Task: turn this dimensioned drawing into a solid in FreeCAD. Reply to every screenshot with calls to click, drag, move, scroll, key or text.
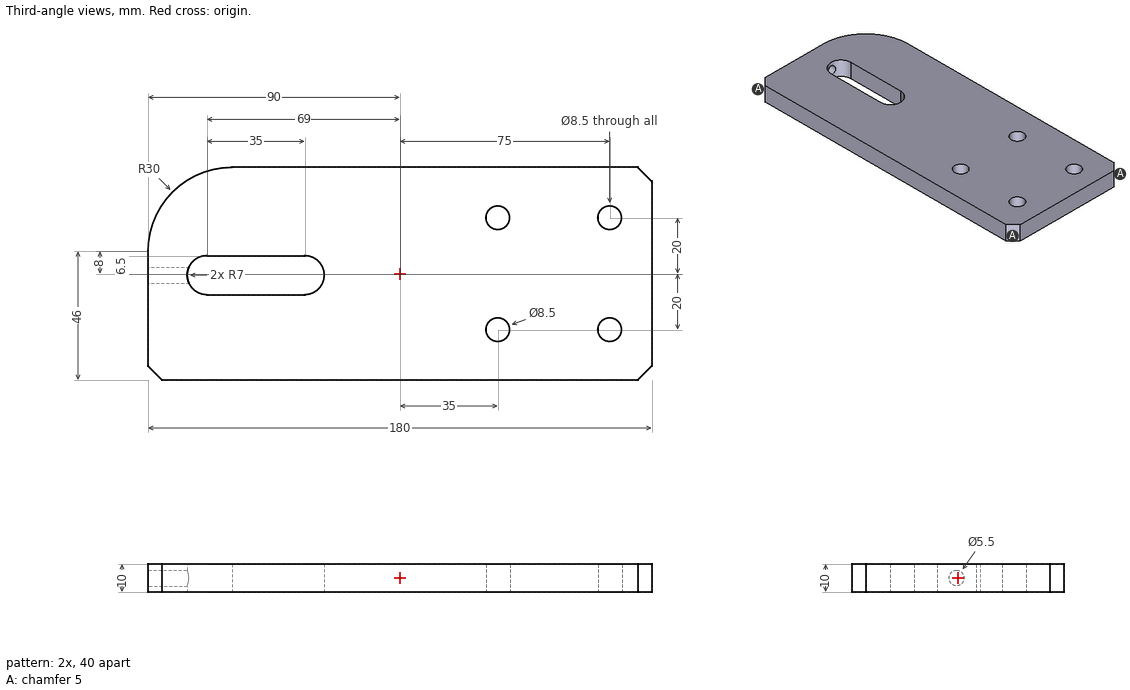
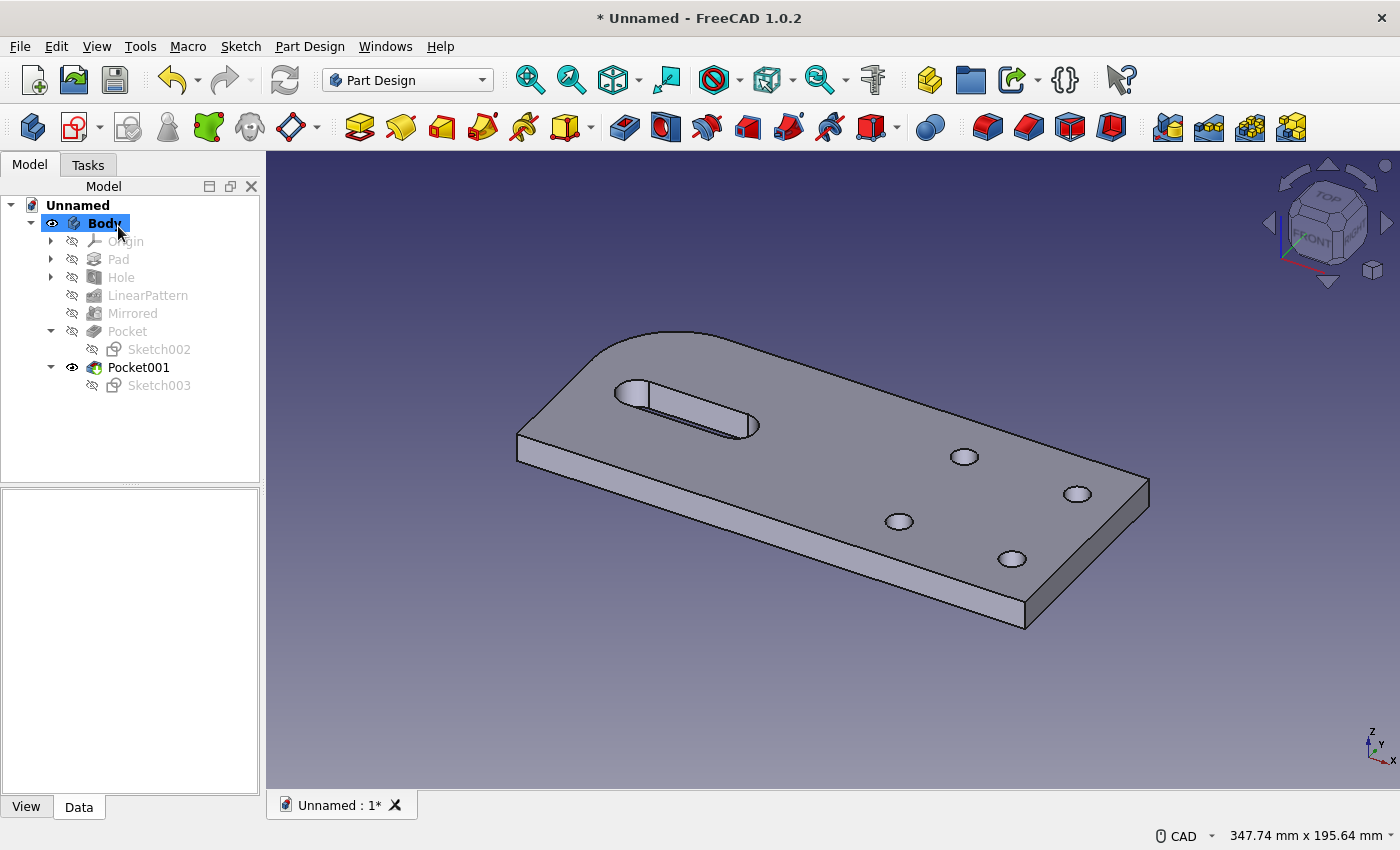
key(6)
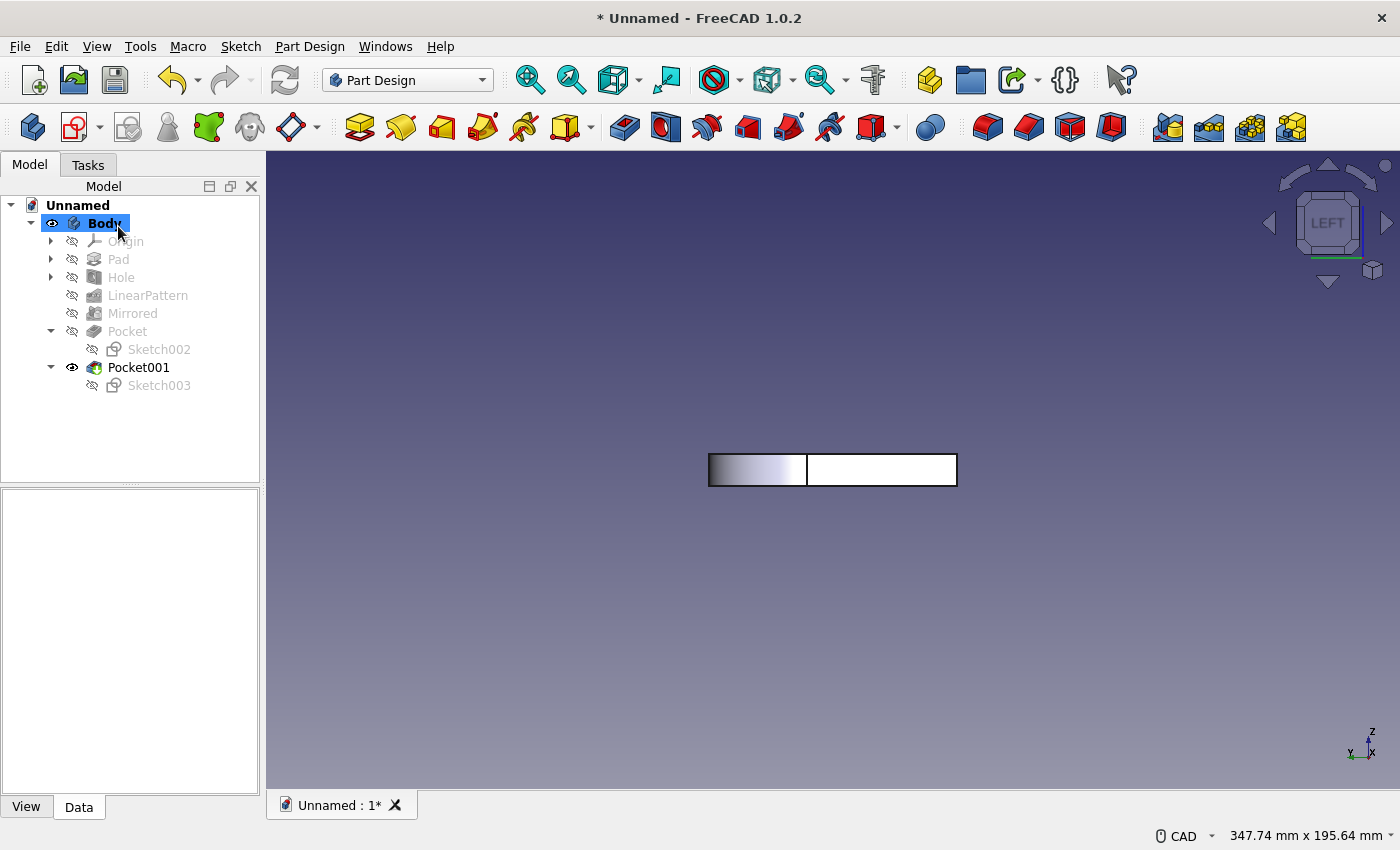
click(531, 80)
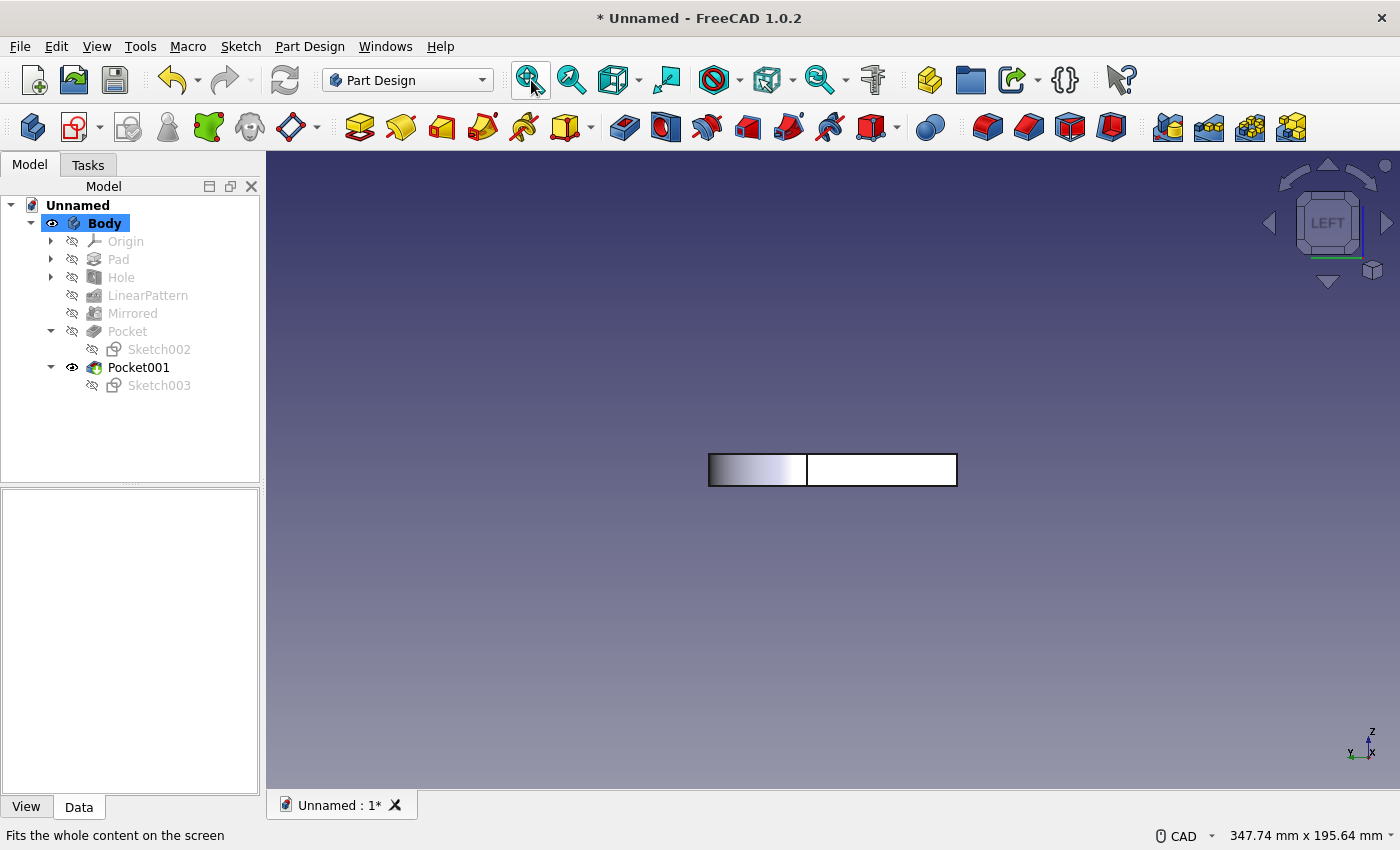
click(839, 469)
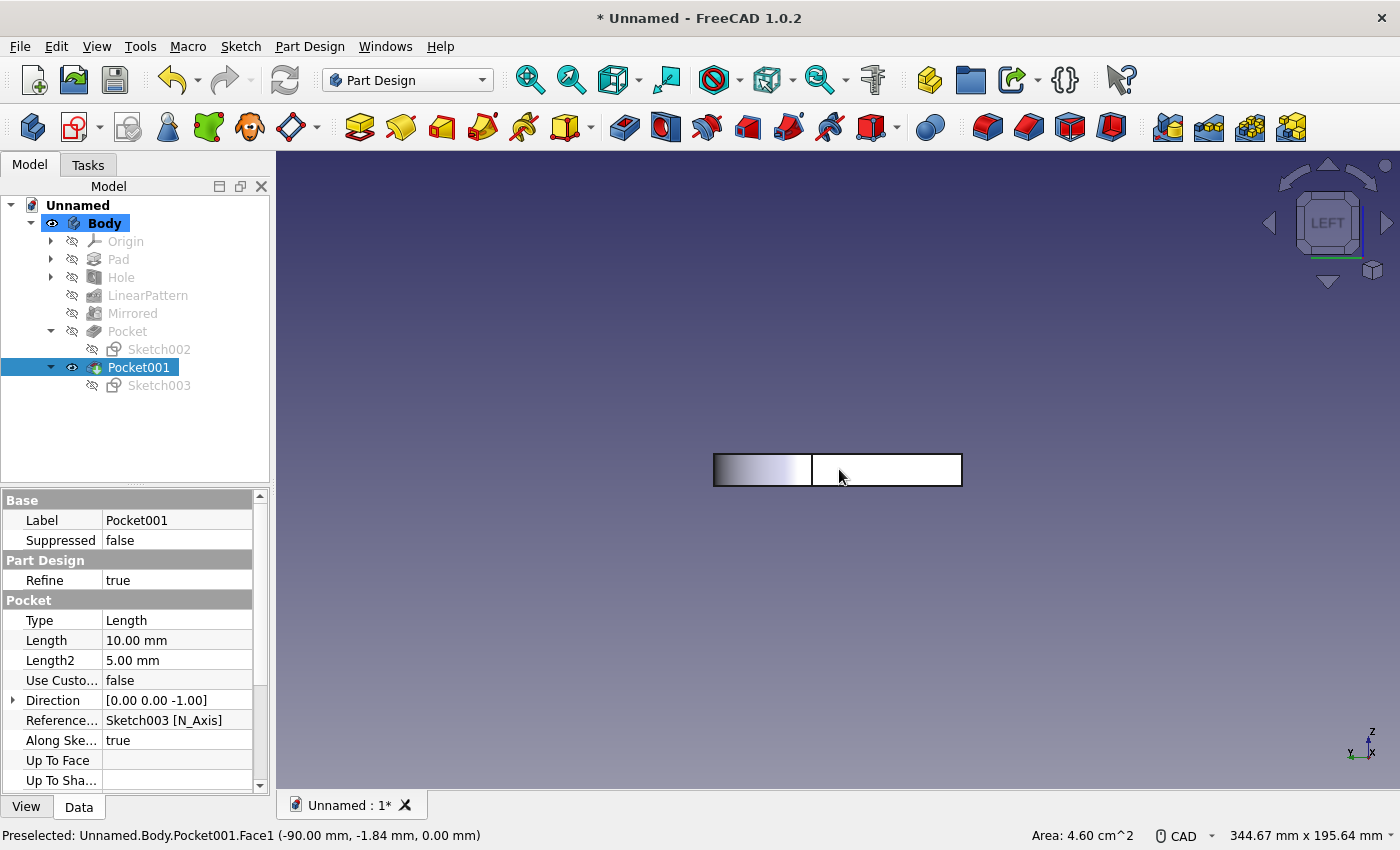
click(74, 128)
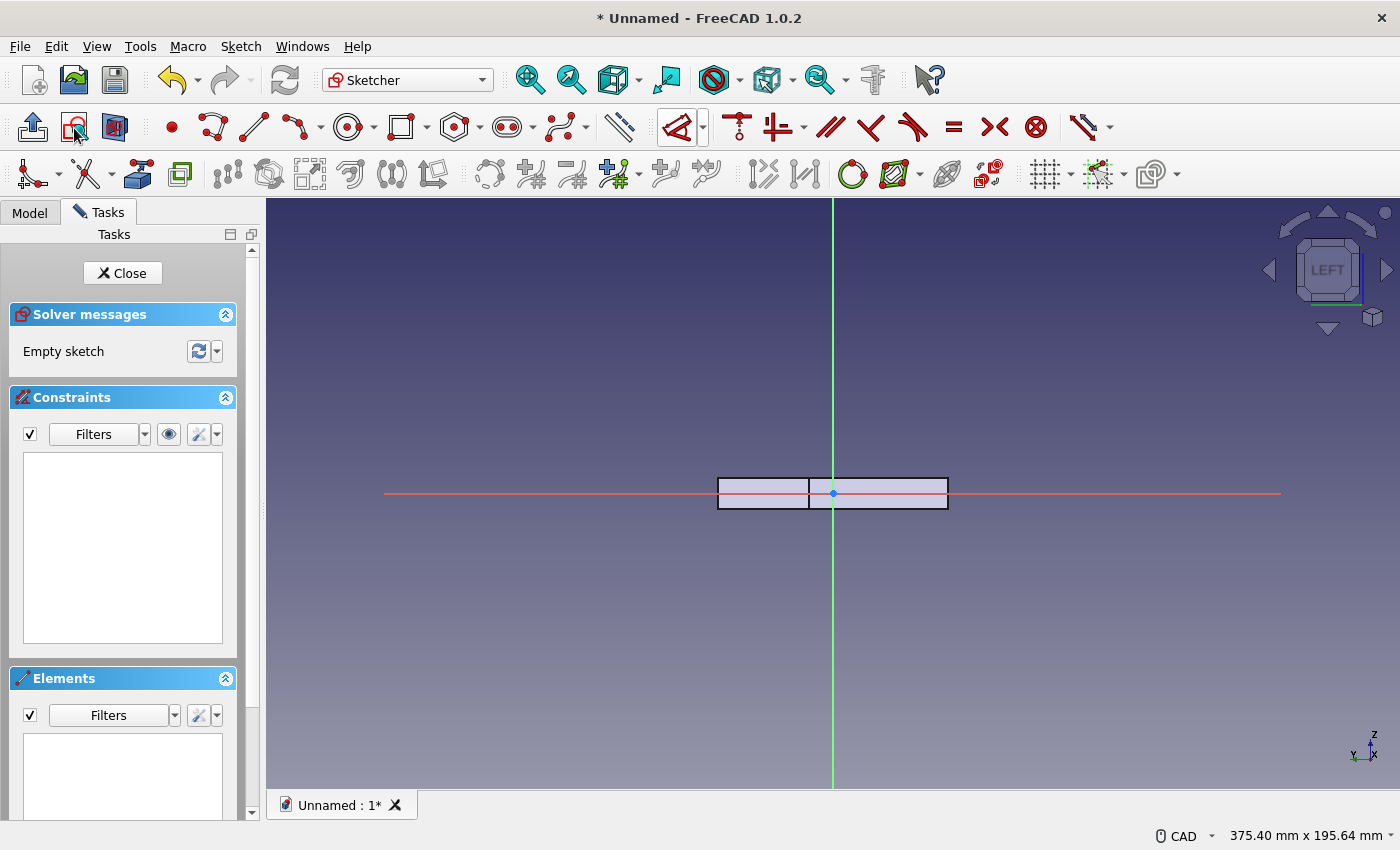
scroll(838, 494, up, 15)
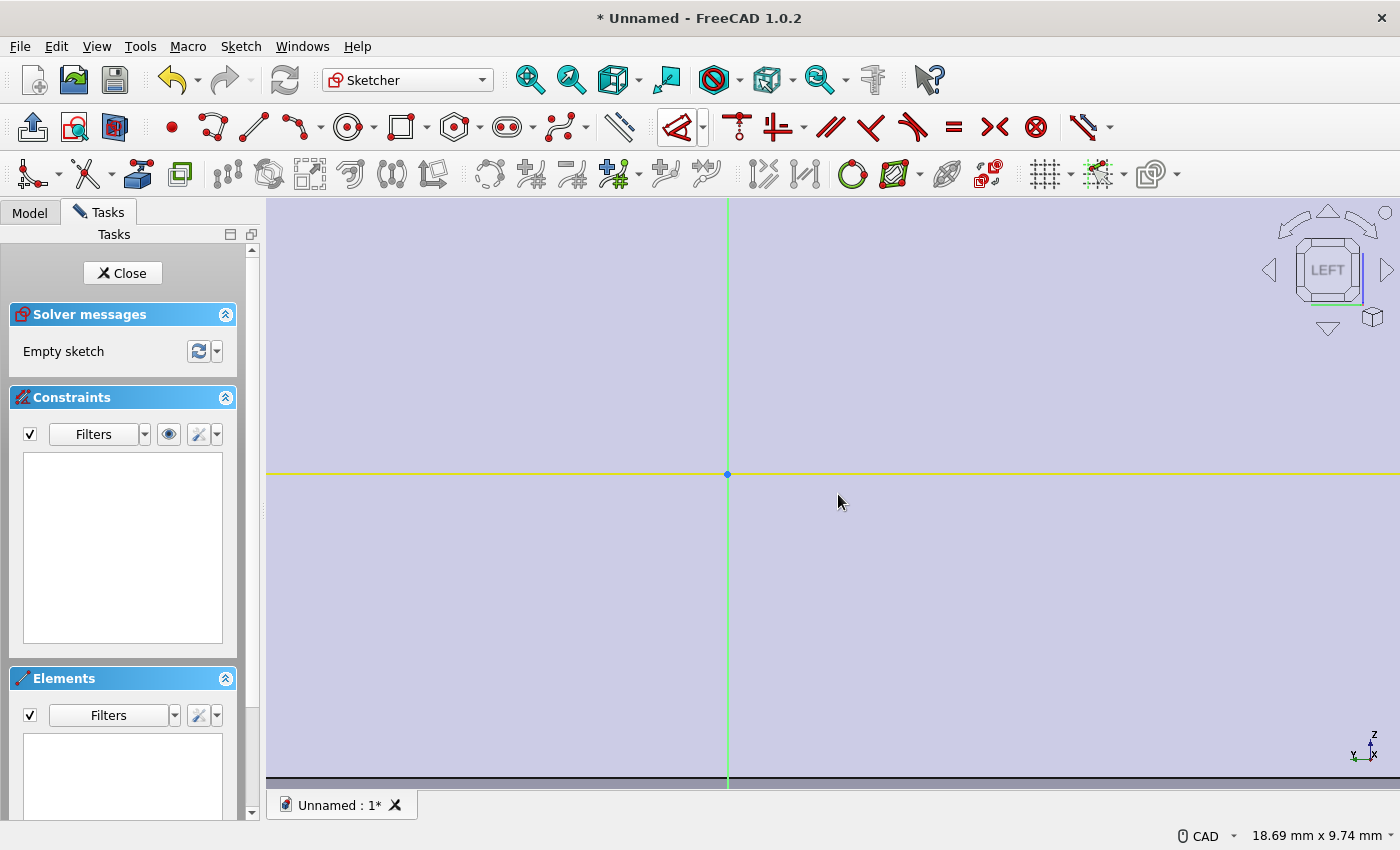
click(348, 128)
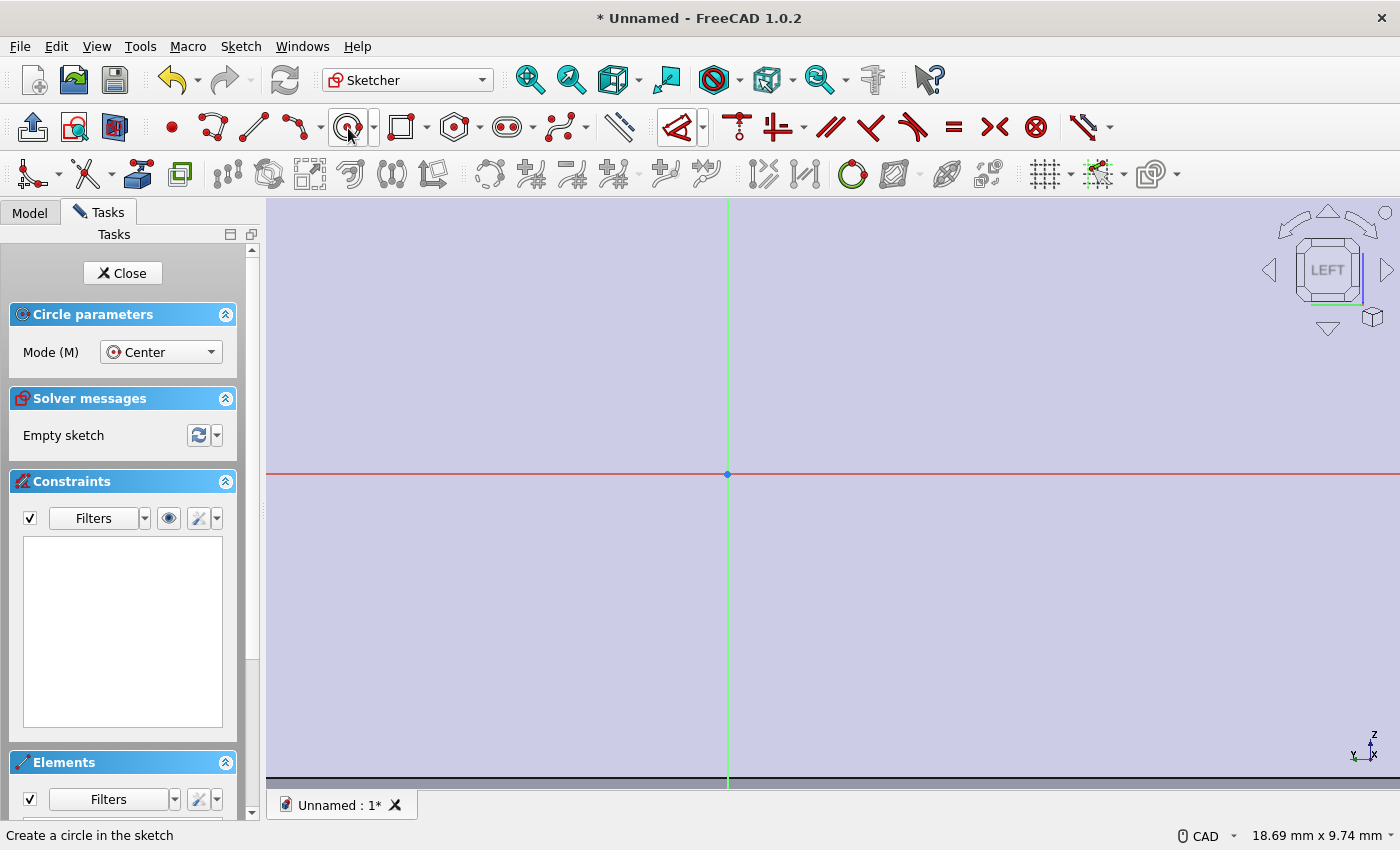
click(758, 474)
click(876, 356)
key(Escape)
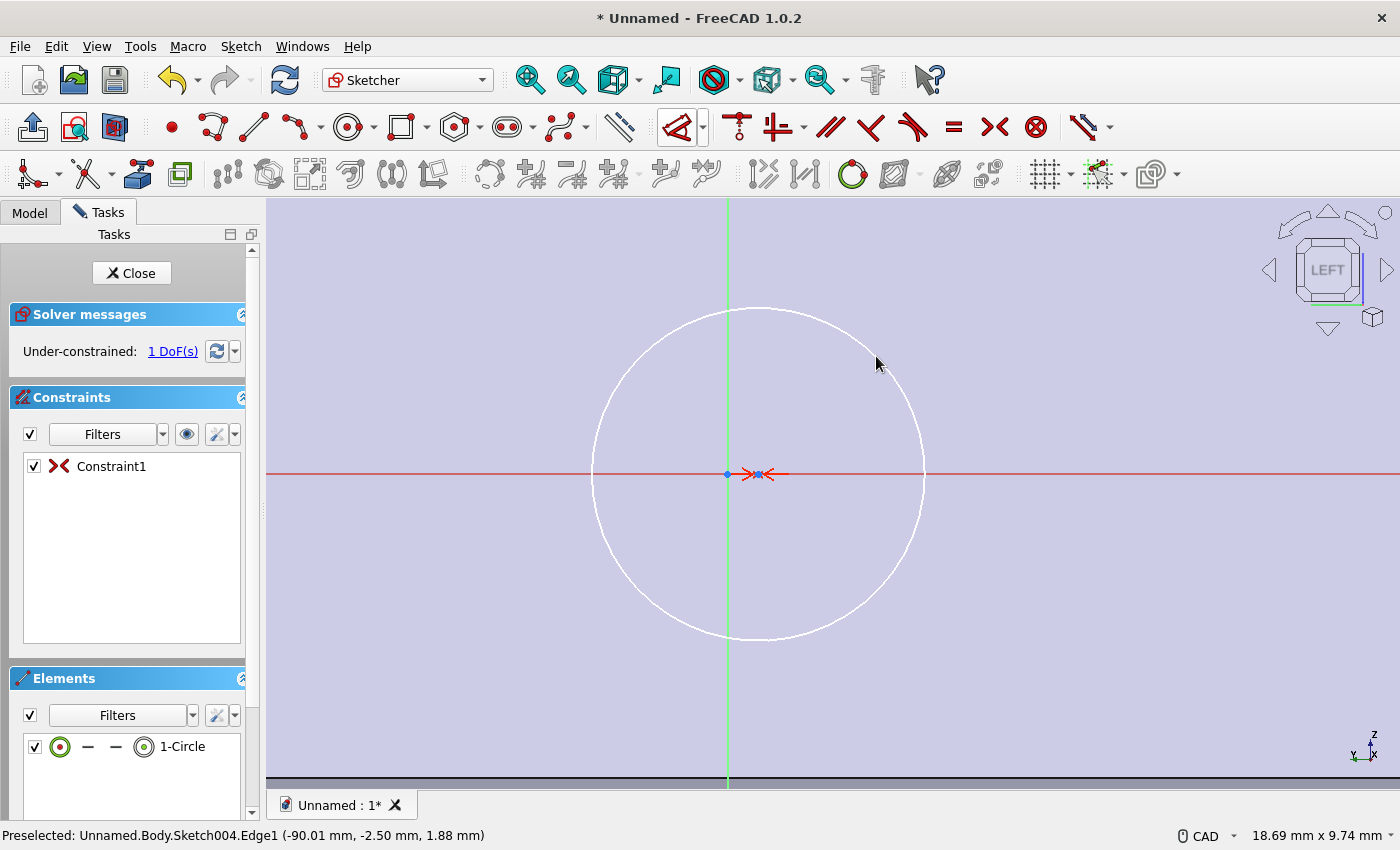
click(876, 356)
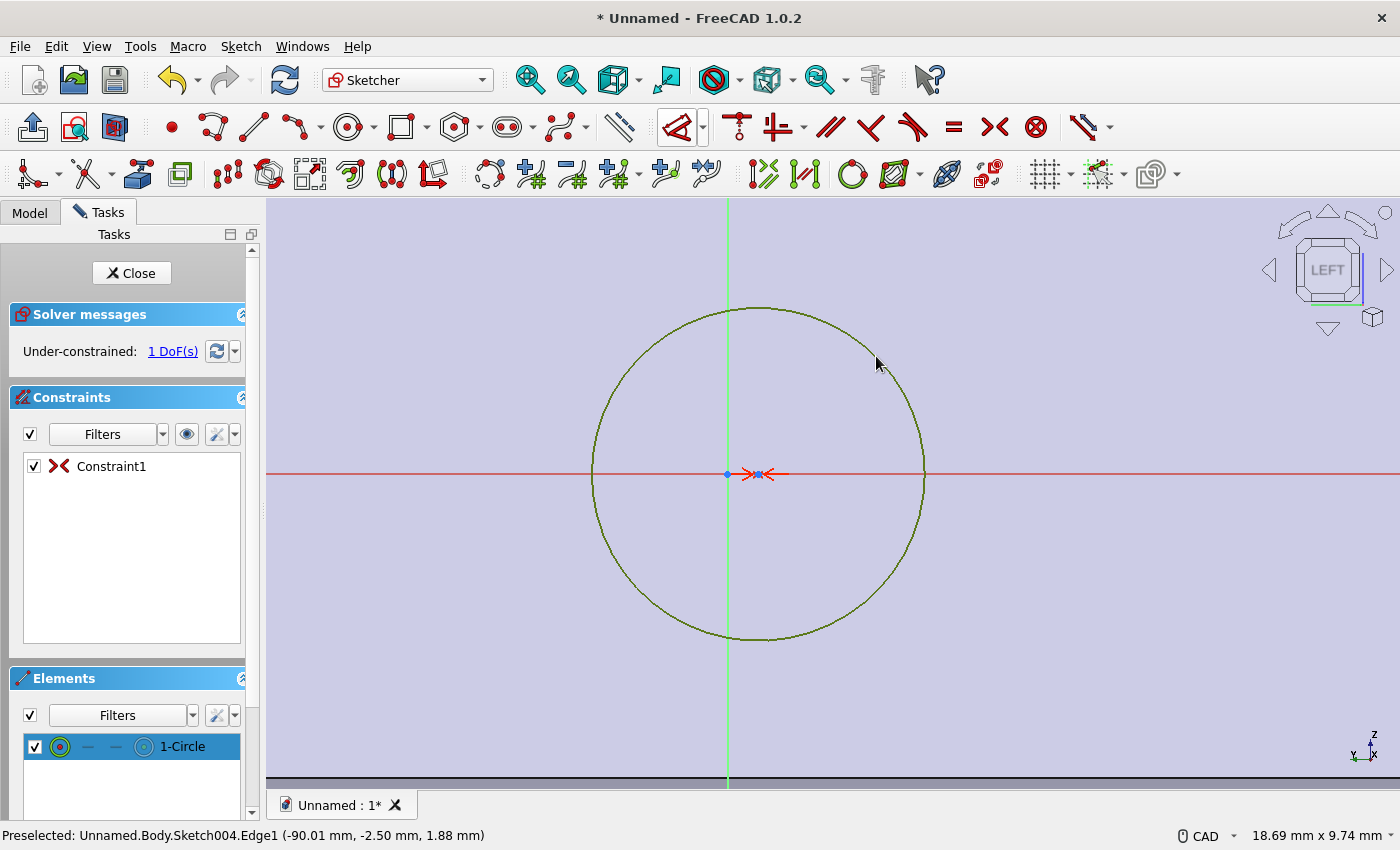
click(702, 128)